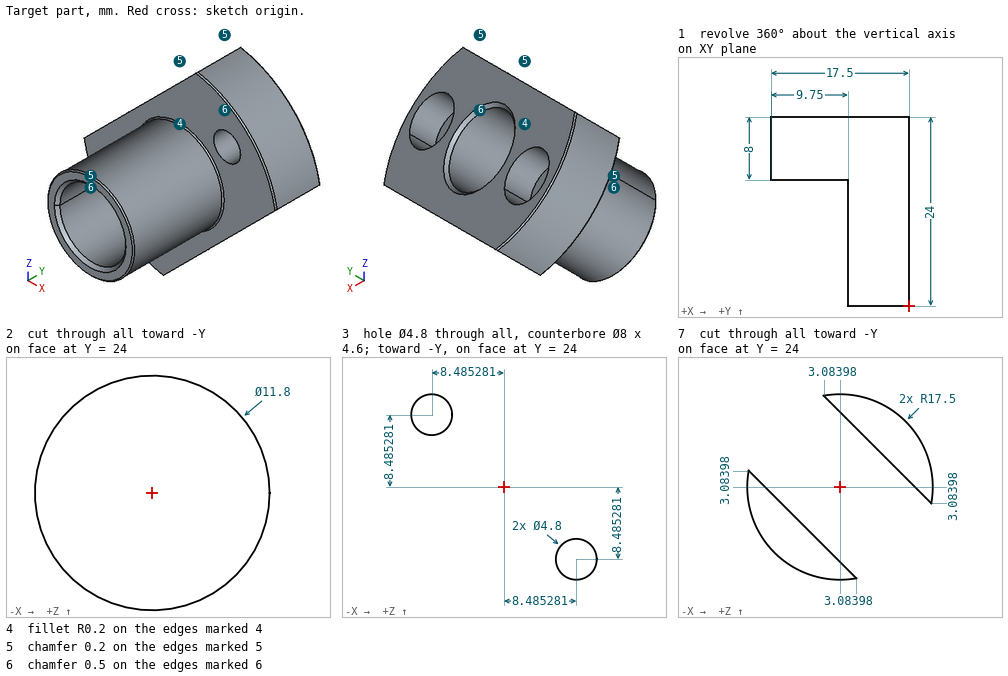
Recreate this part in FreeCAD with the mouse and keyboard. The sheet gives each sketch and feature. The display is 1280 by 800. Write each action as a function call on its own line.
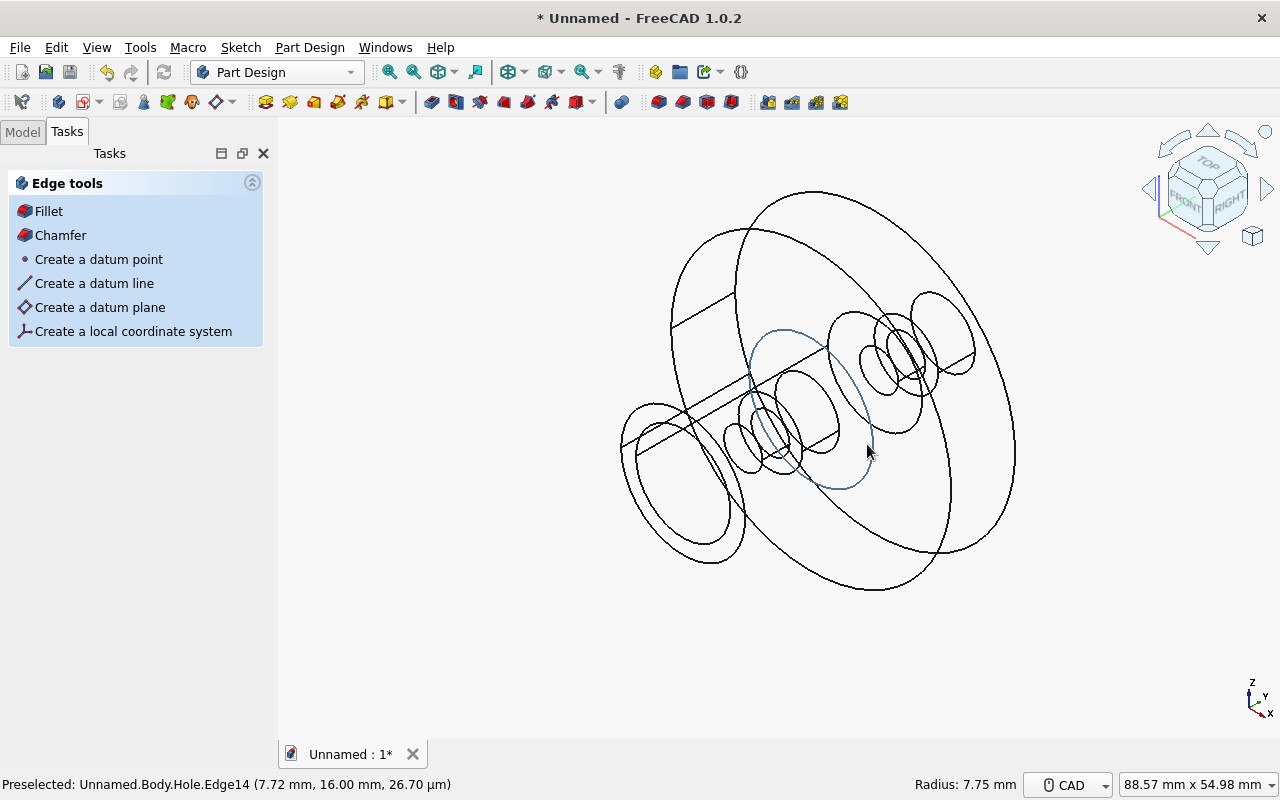
key(v)
key(1)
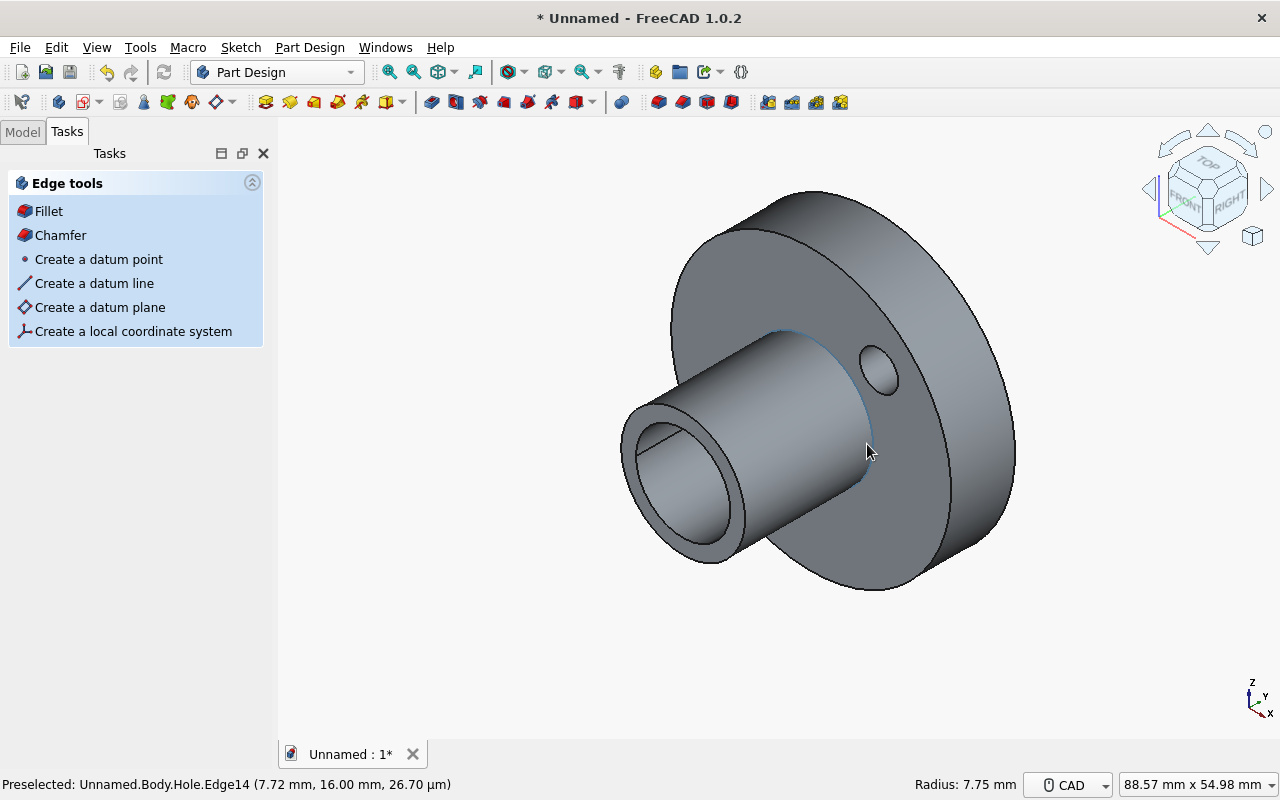
click(660, 102)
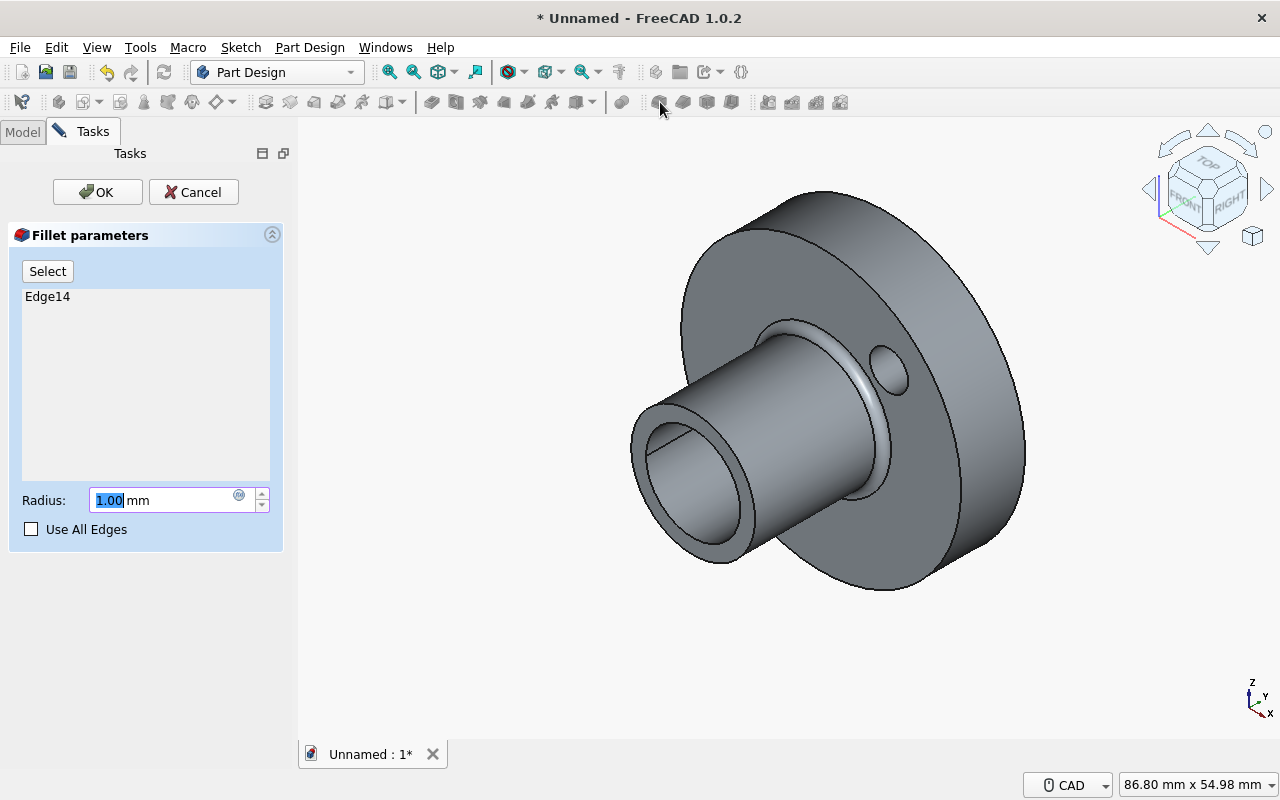
text(0.2)
key(Tab)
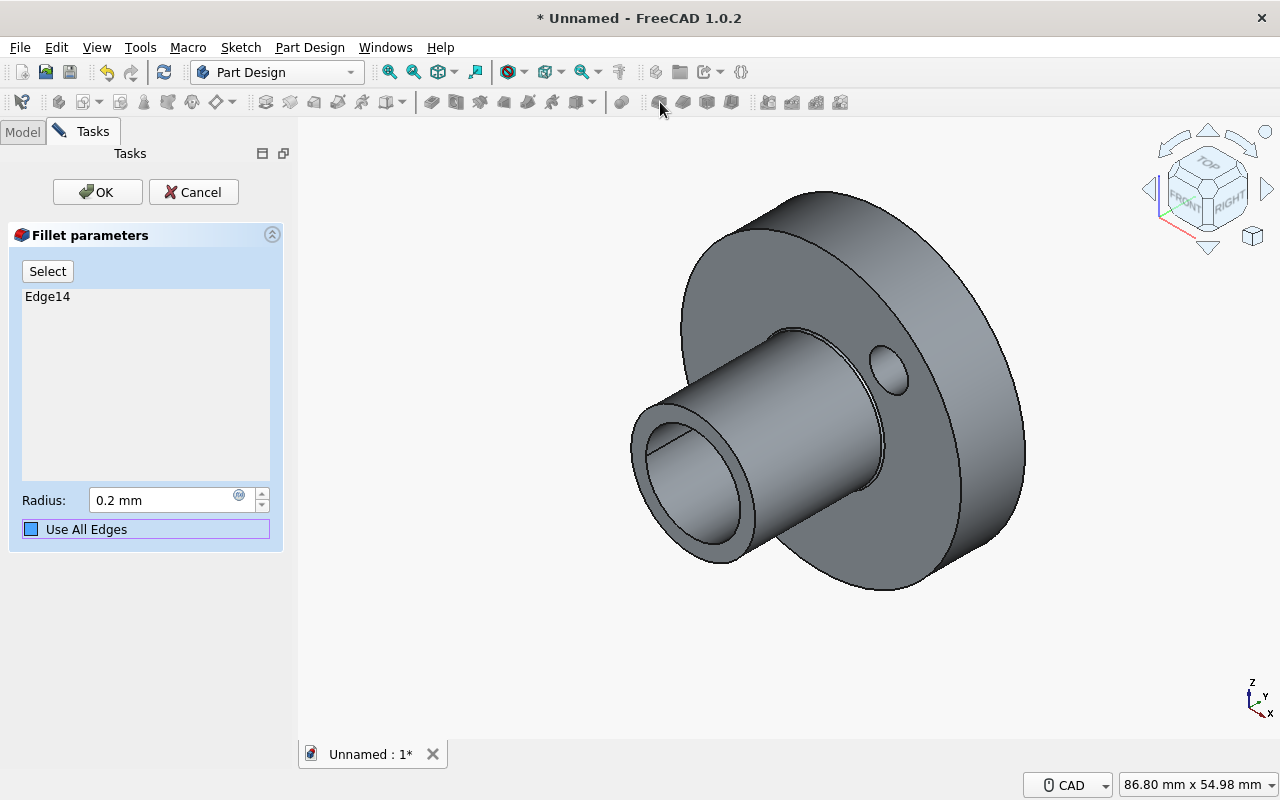
click(98, 192)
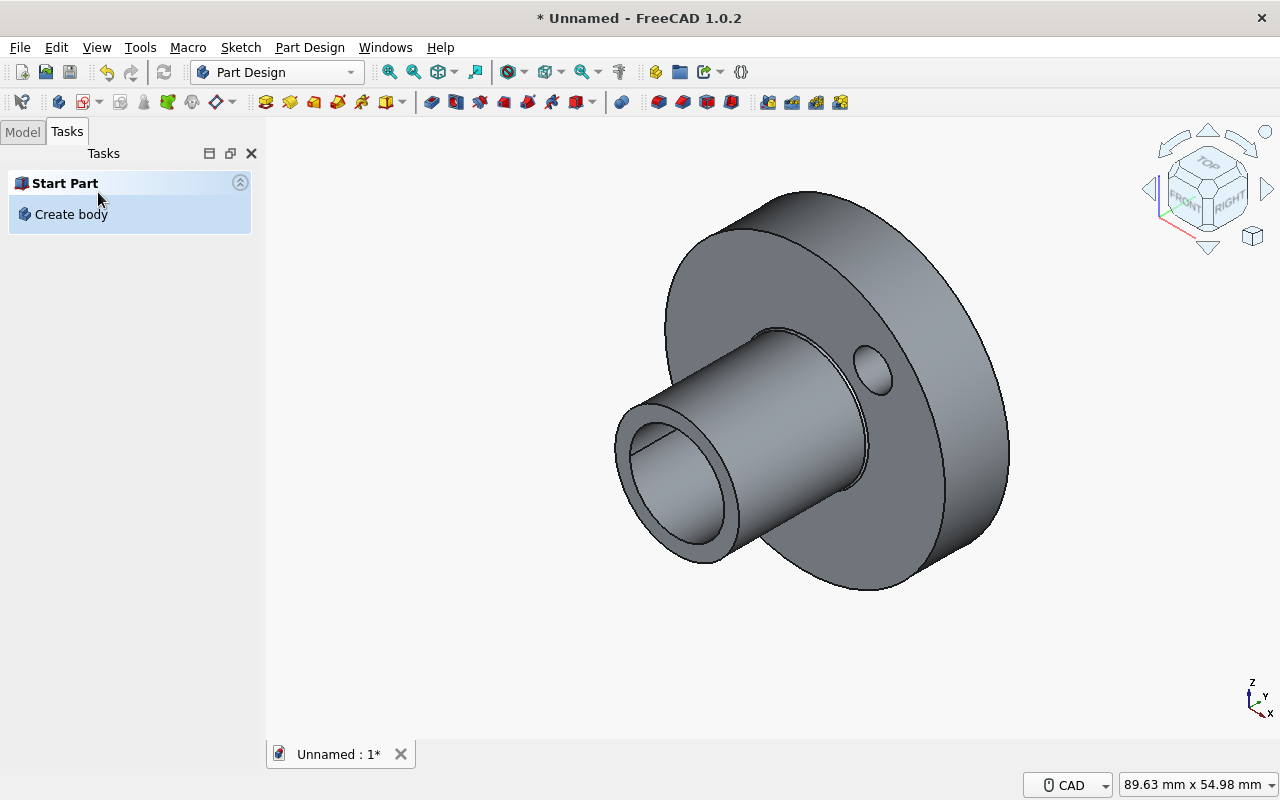
click(739, 518)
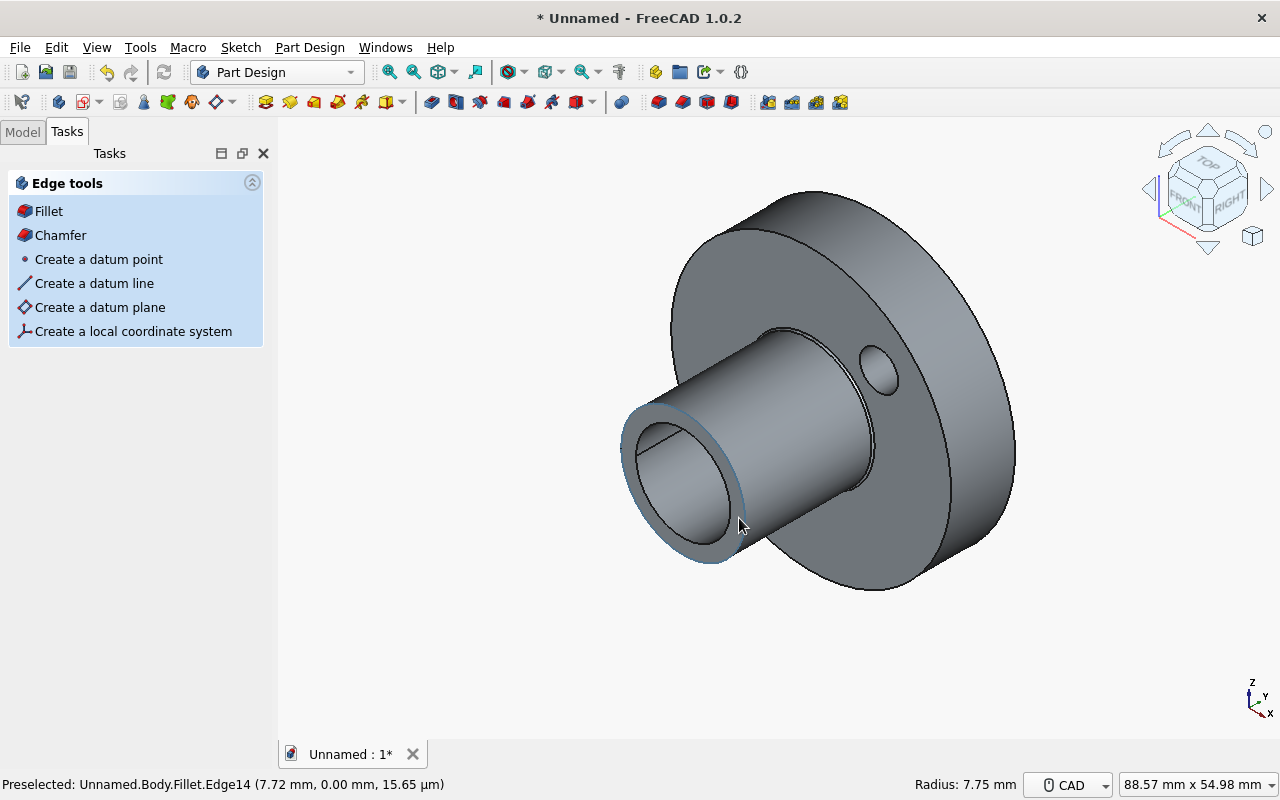
click(951, 489, ctrl)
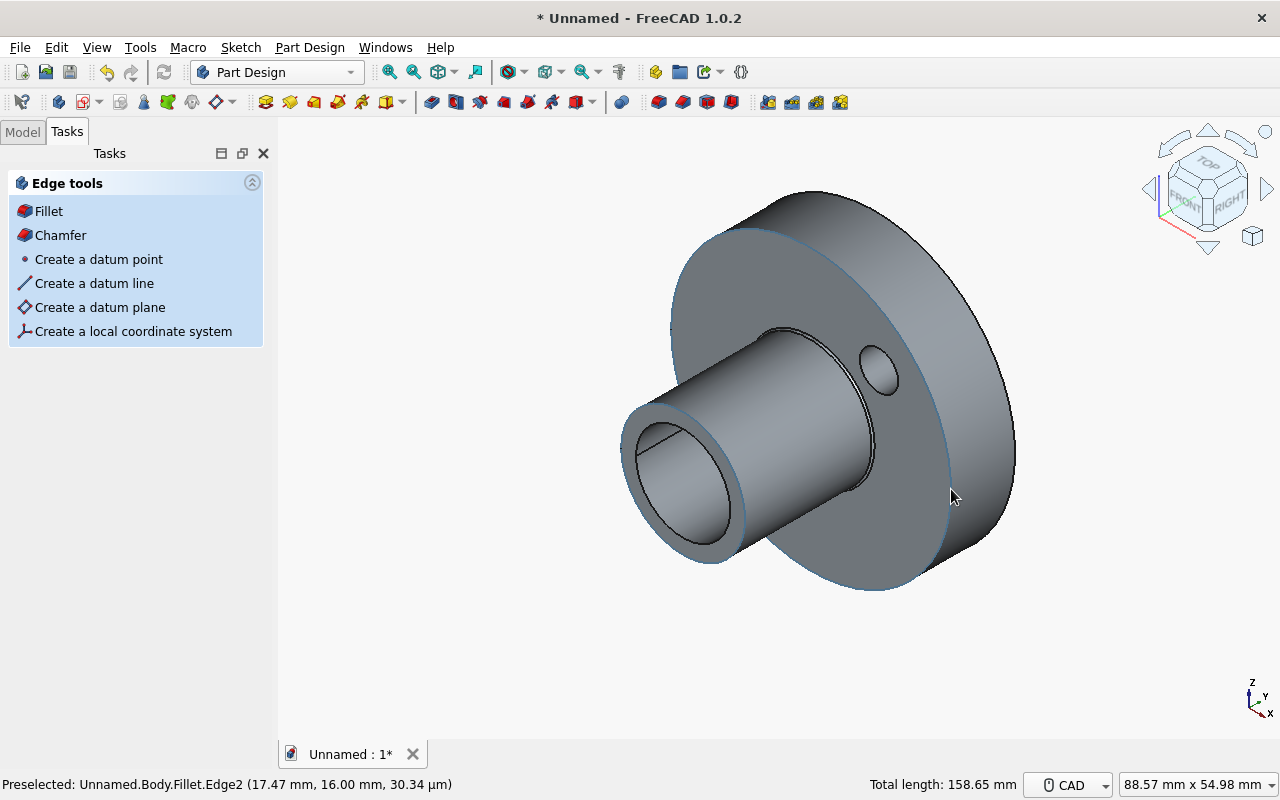
key(2)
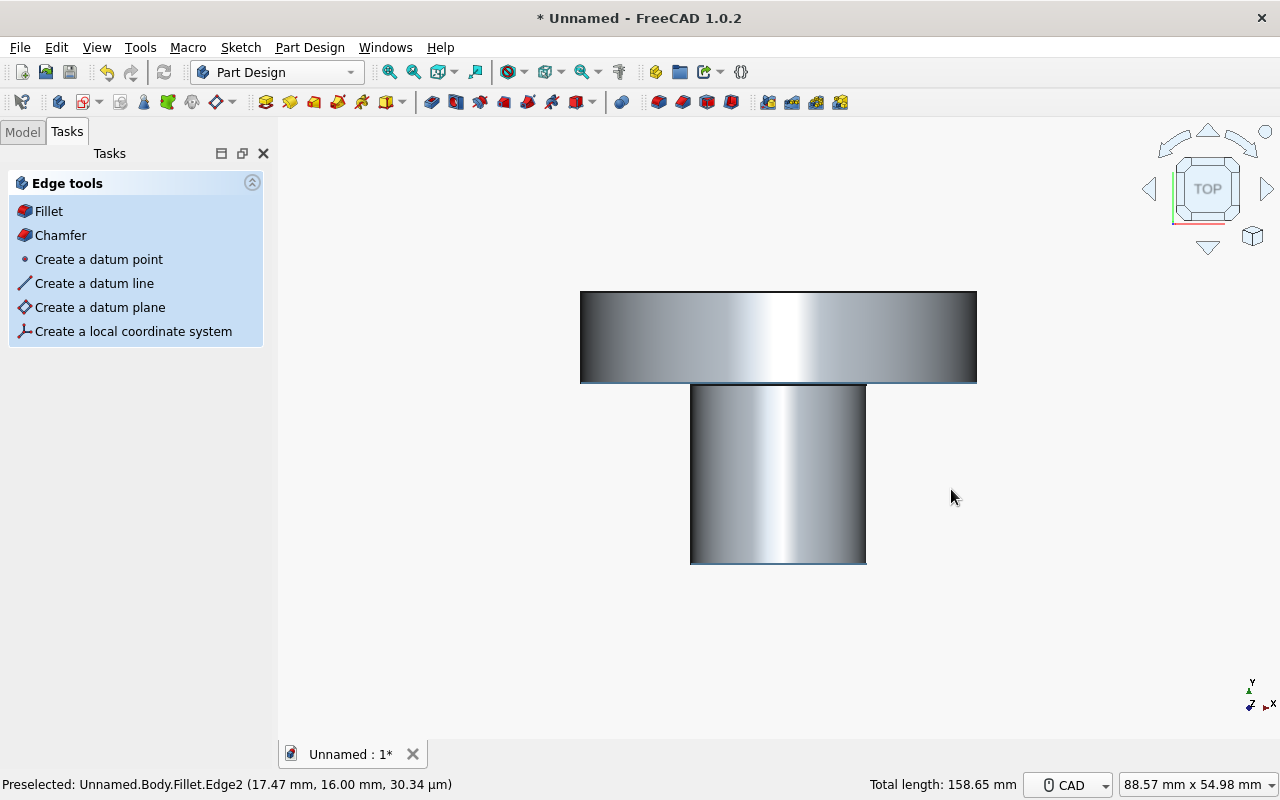
key(v)
key(f)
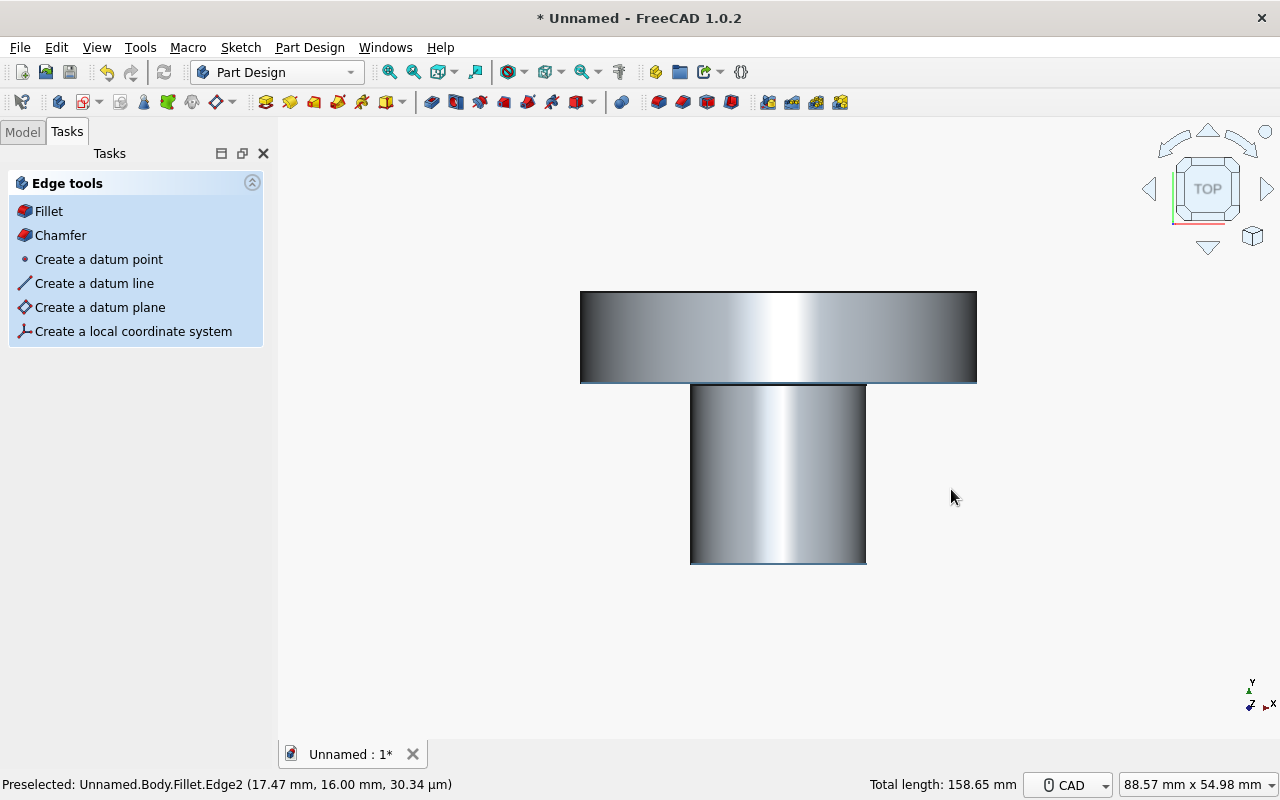
click(939, 291, ctrl)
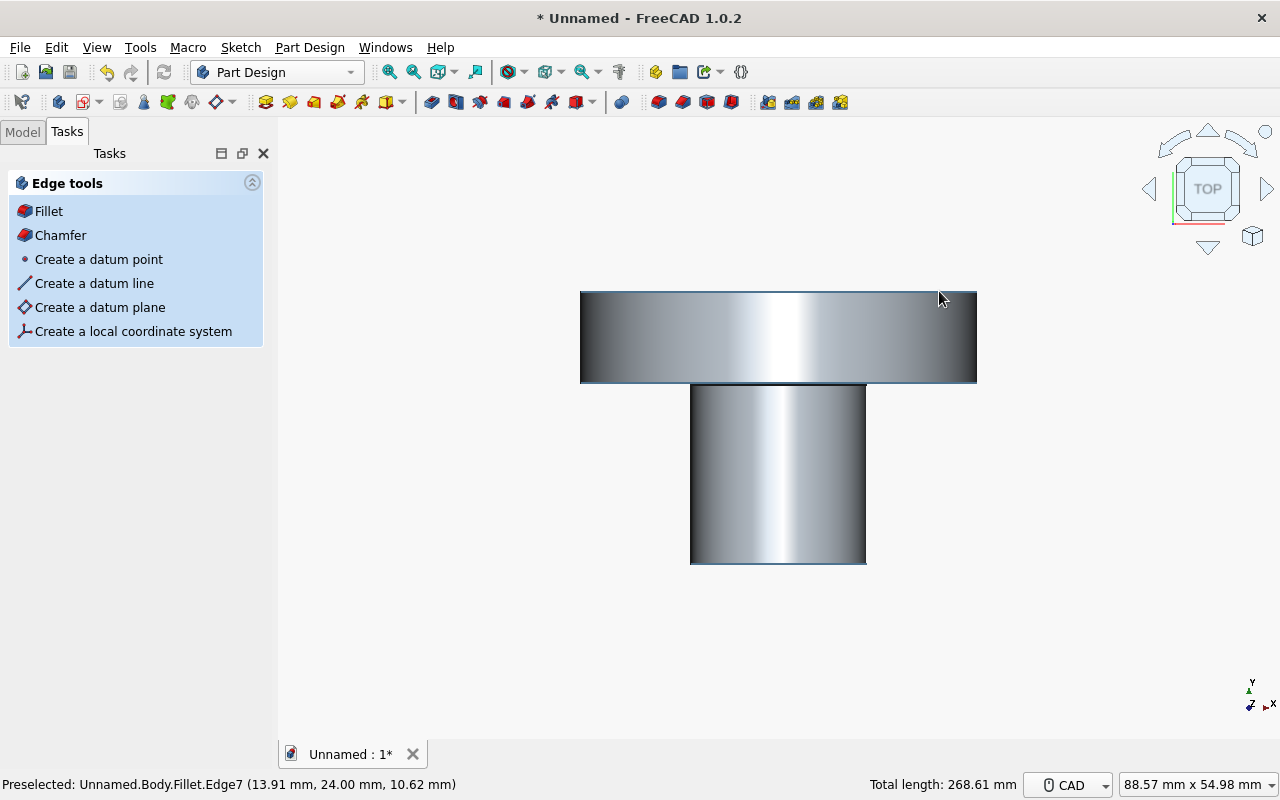
click(684, 102)